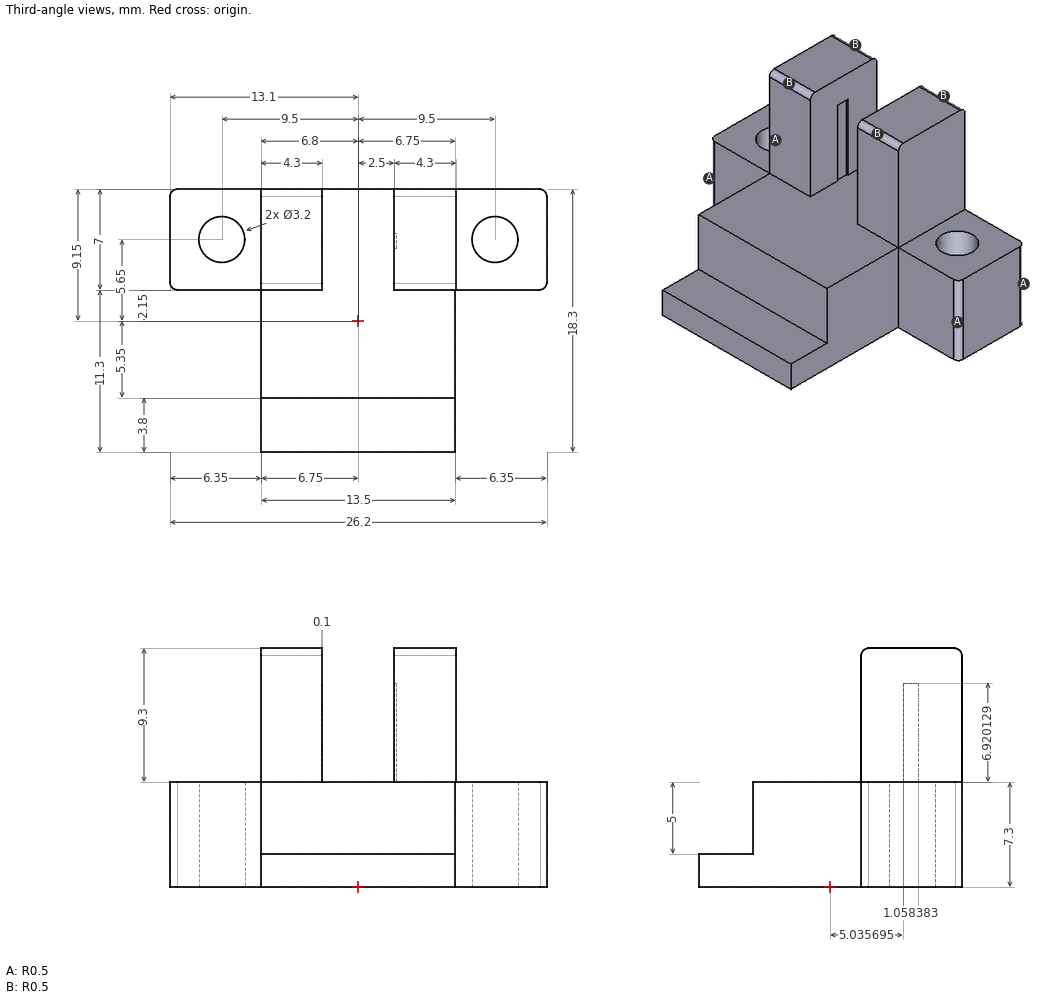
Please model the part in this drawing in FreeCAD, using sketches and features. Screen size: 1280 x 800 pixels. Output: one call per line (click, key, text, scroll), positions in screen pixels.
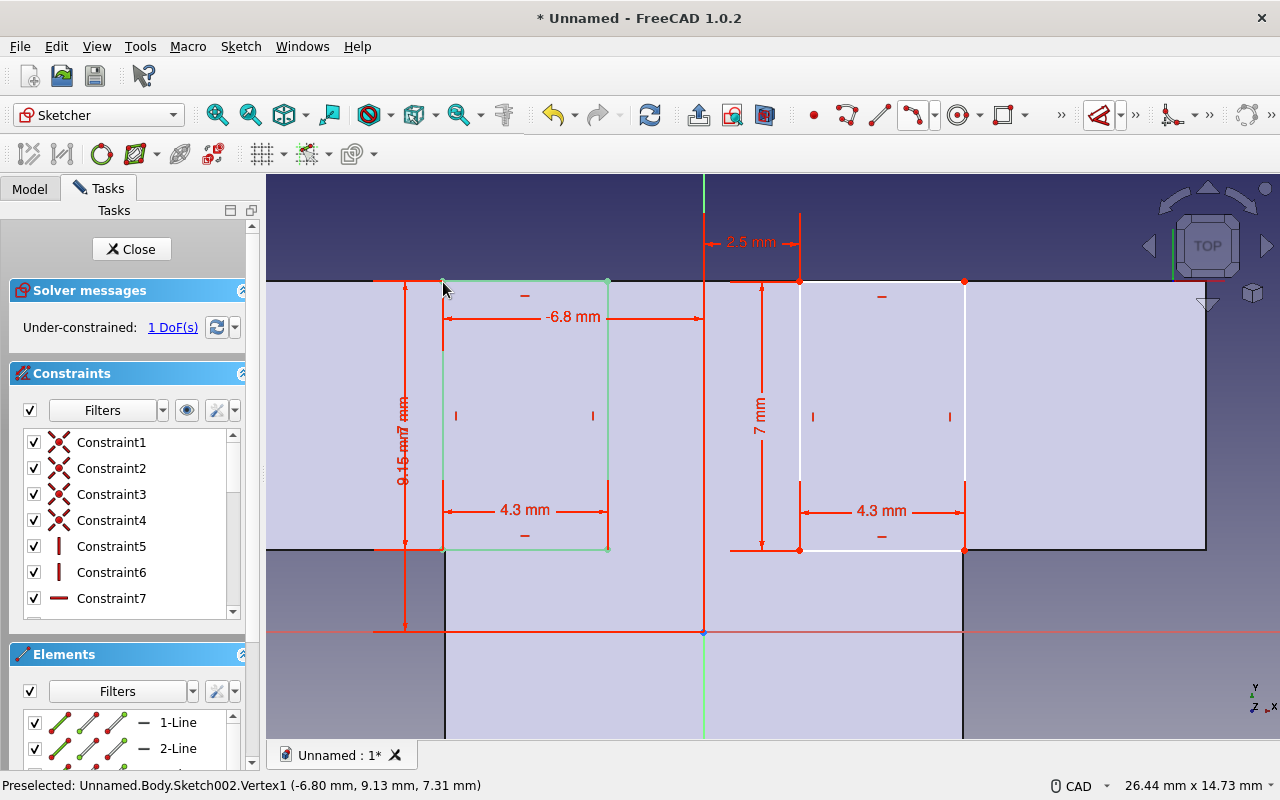
click(800, 282)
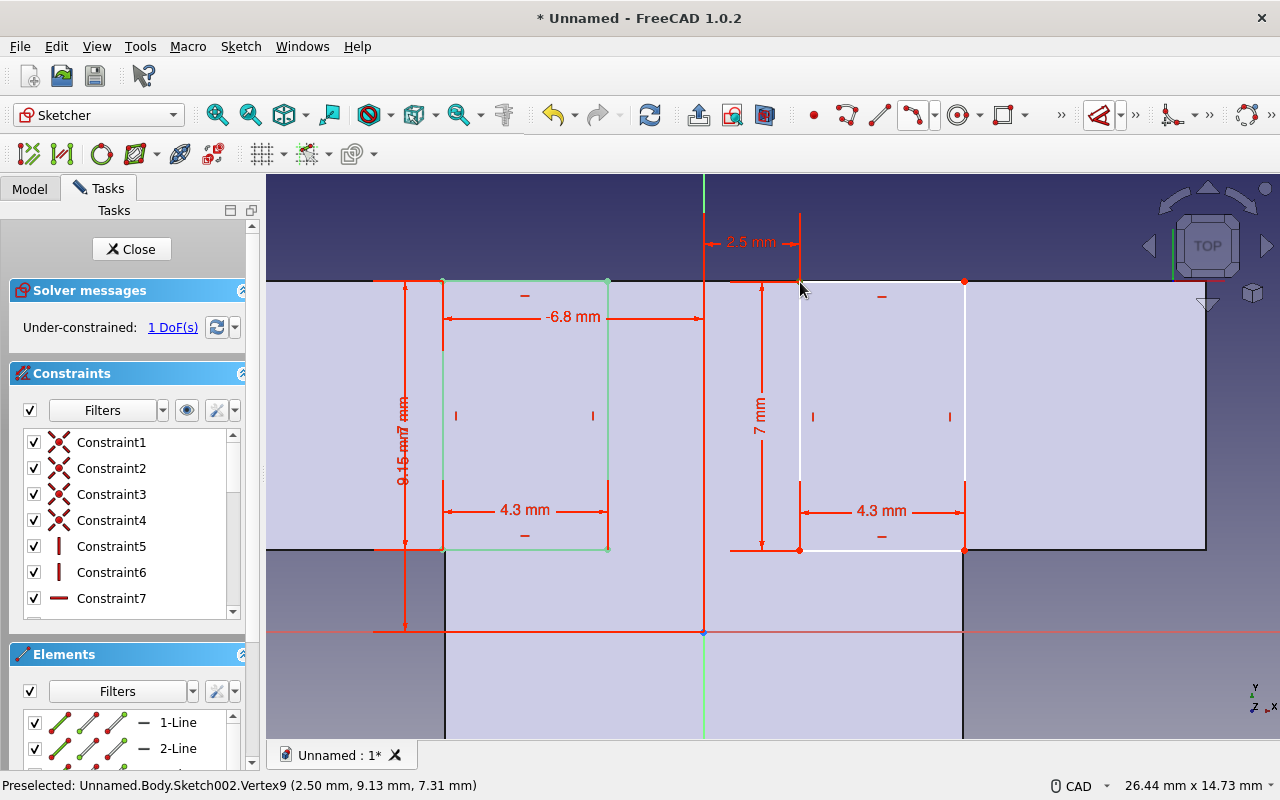
key(i)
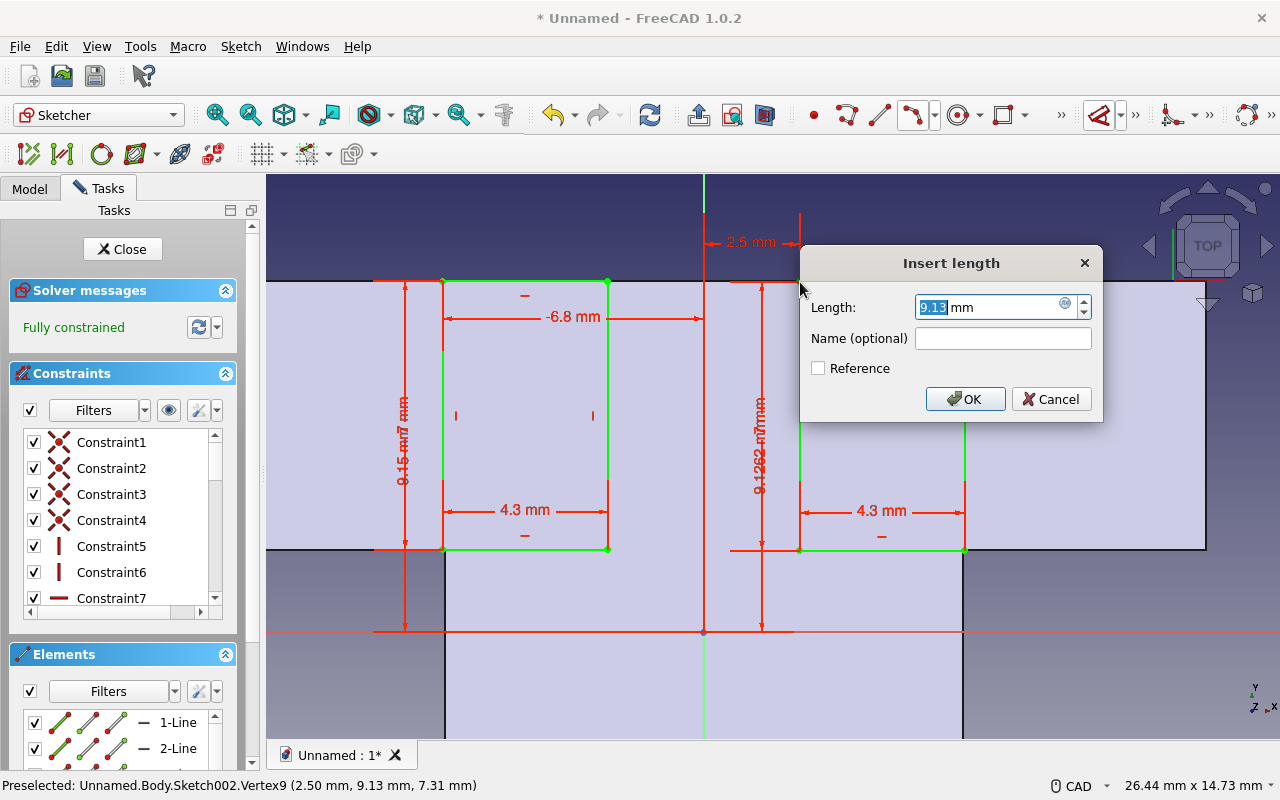
text(9.15)
key(Return)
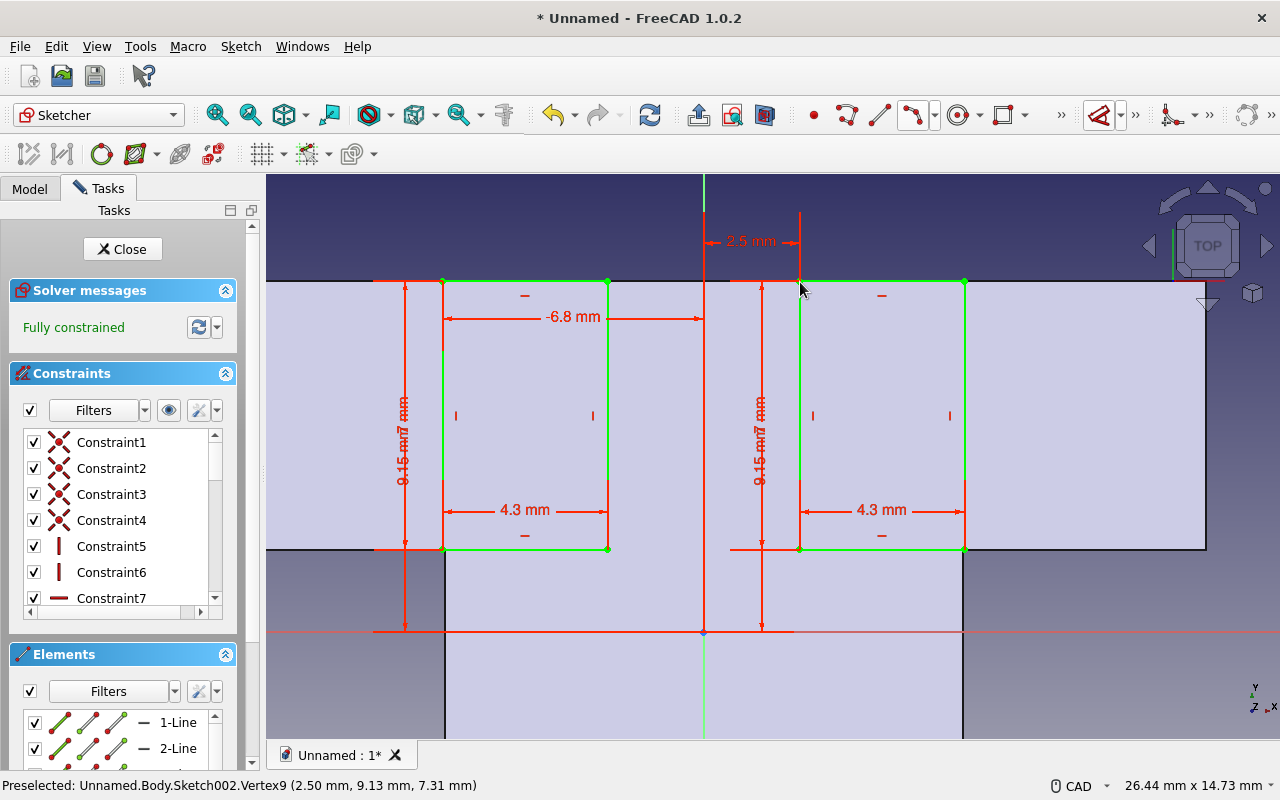
click(123, 249)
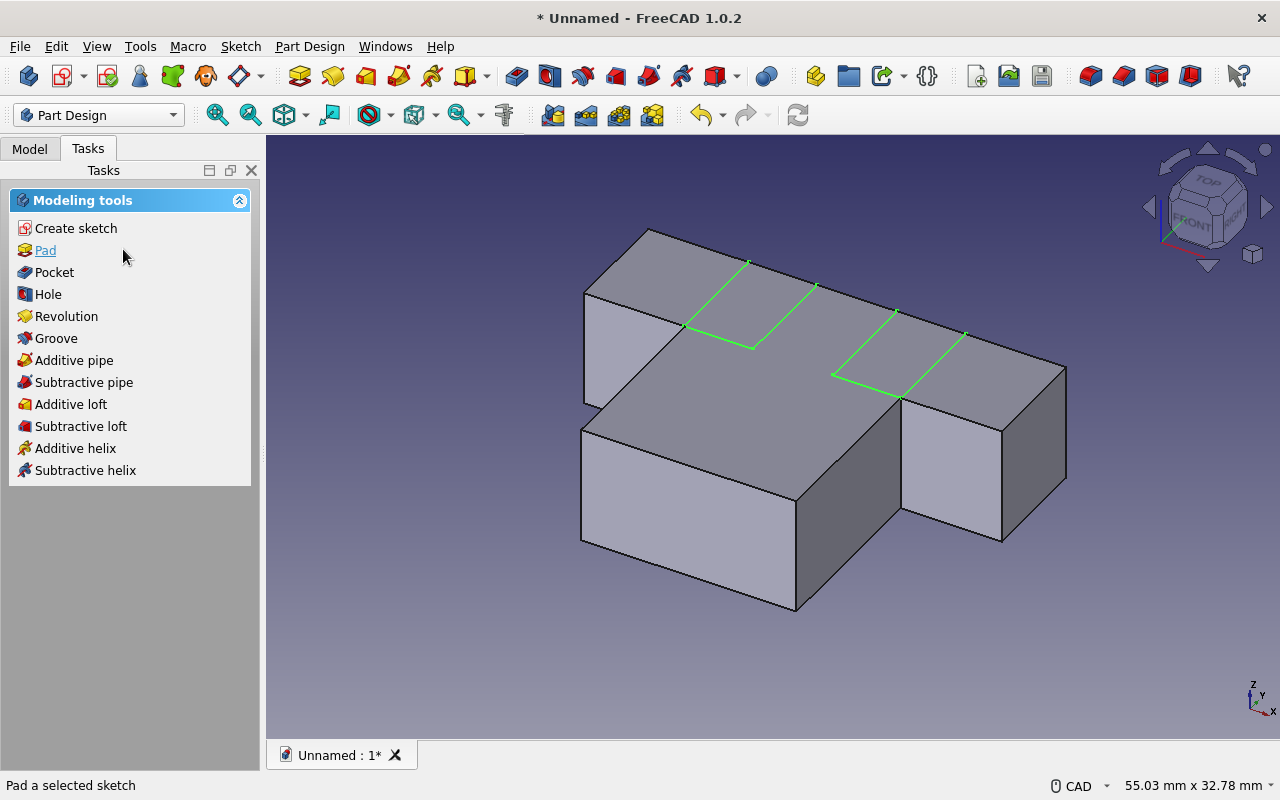
click(300, 76)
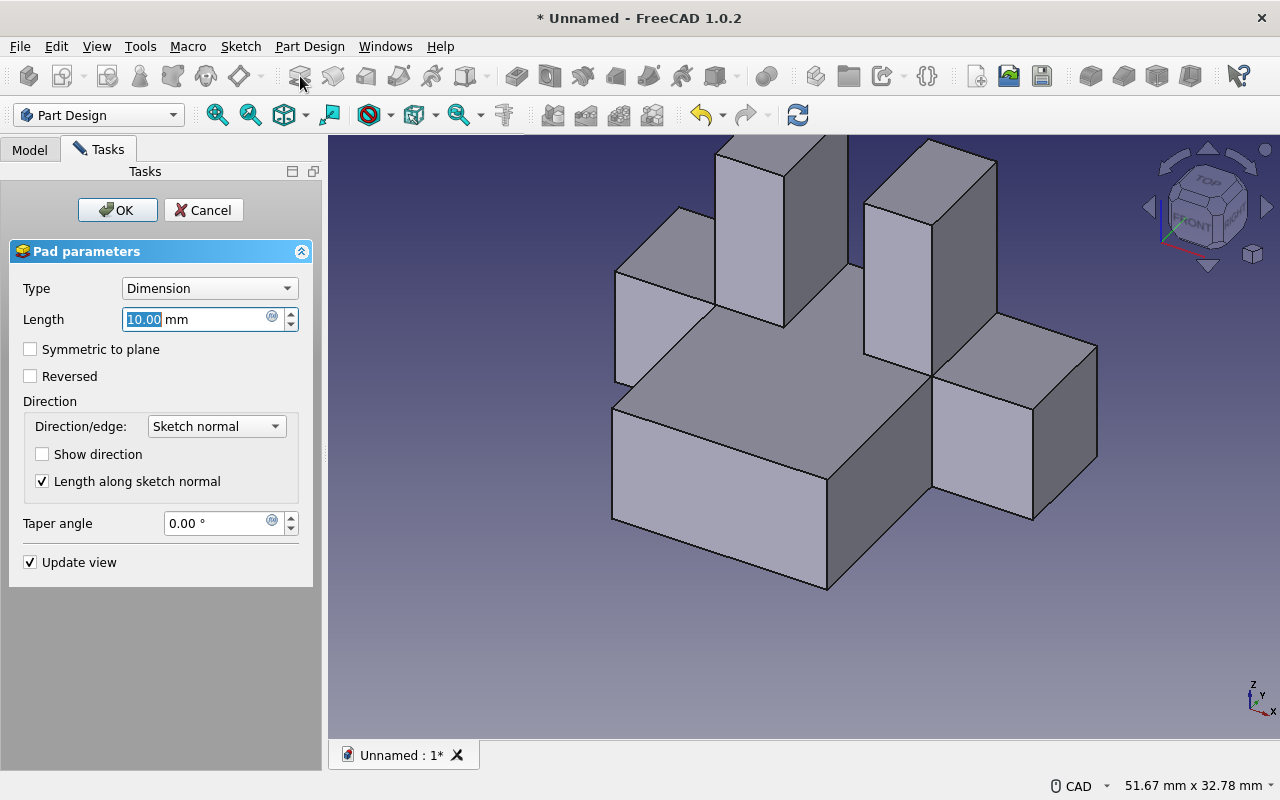
text(9.3)
key(Tab)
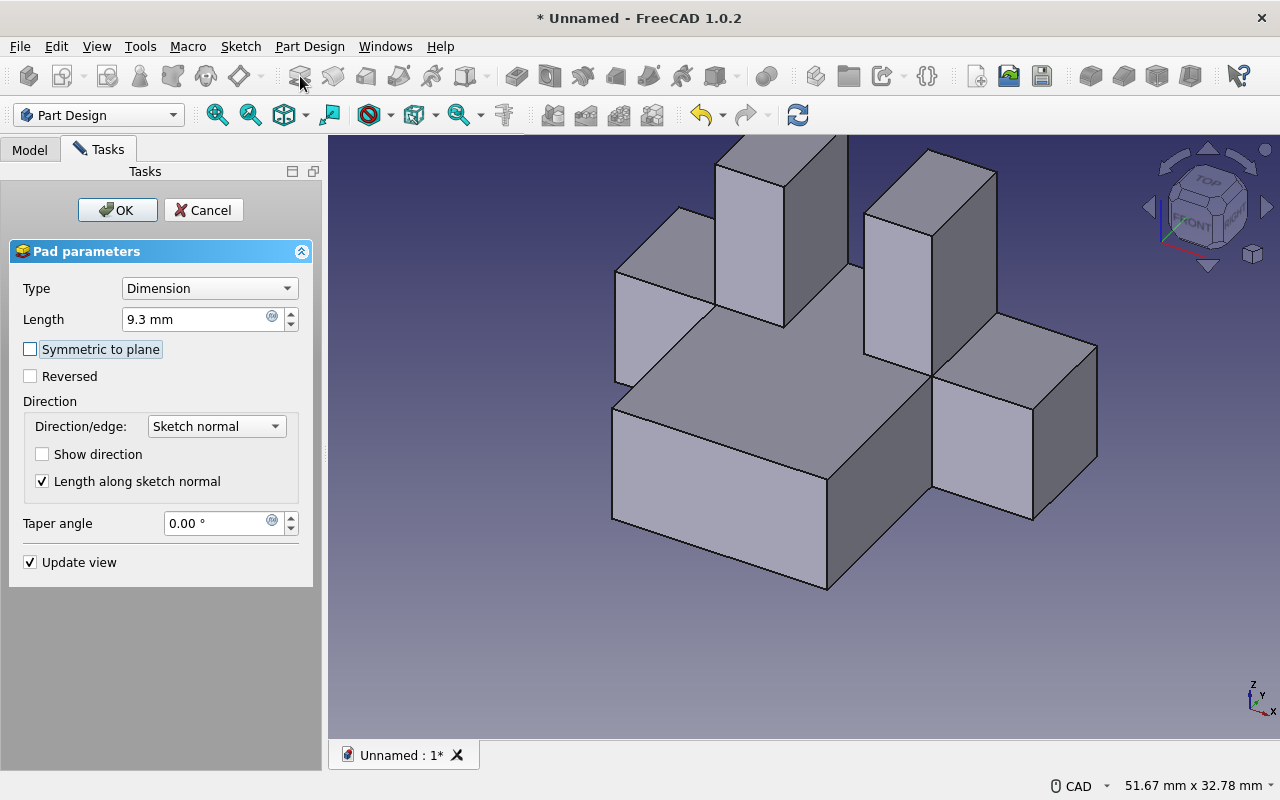
click(118, 210)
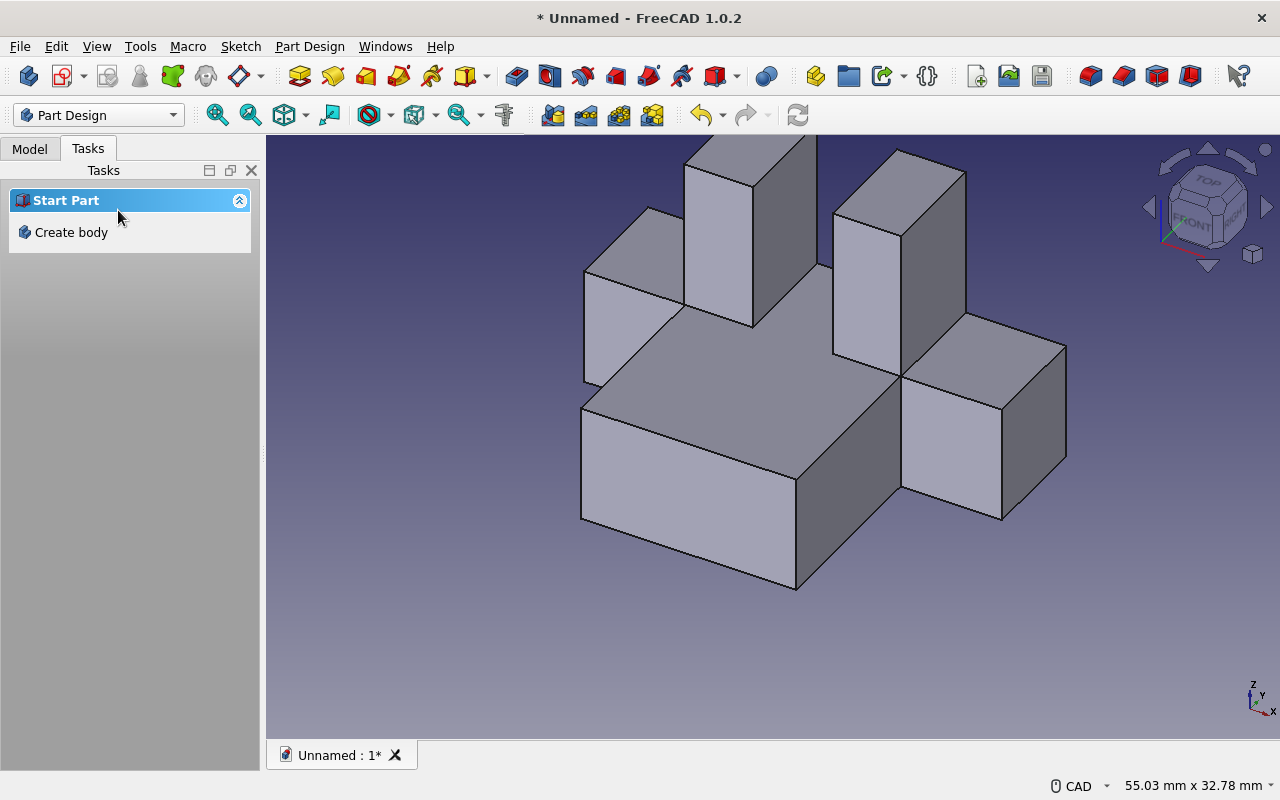
click(218, 116)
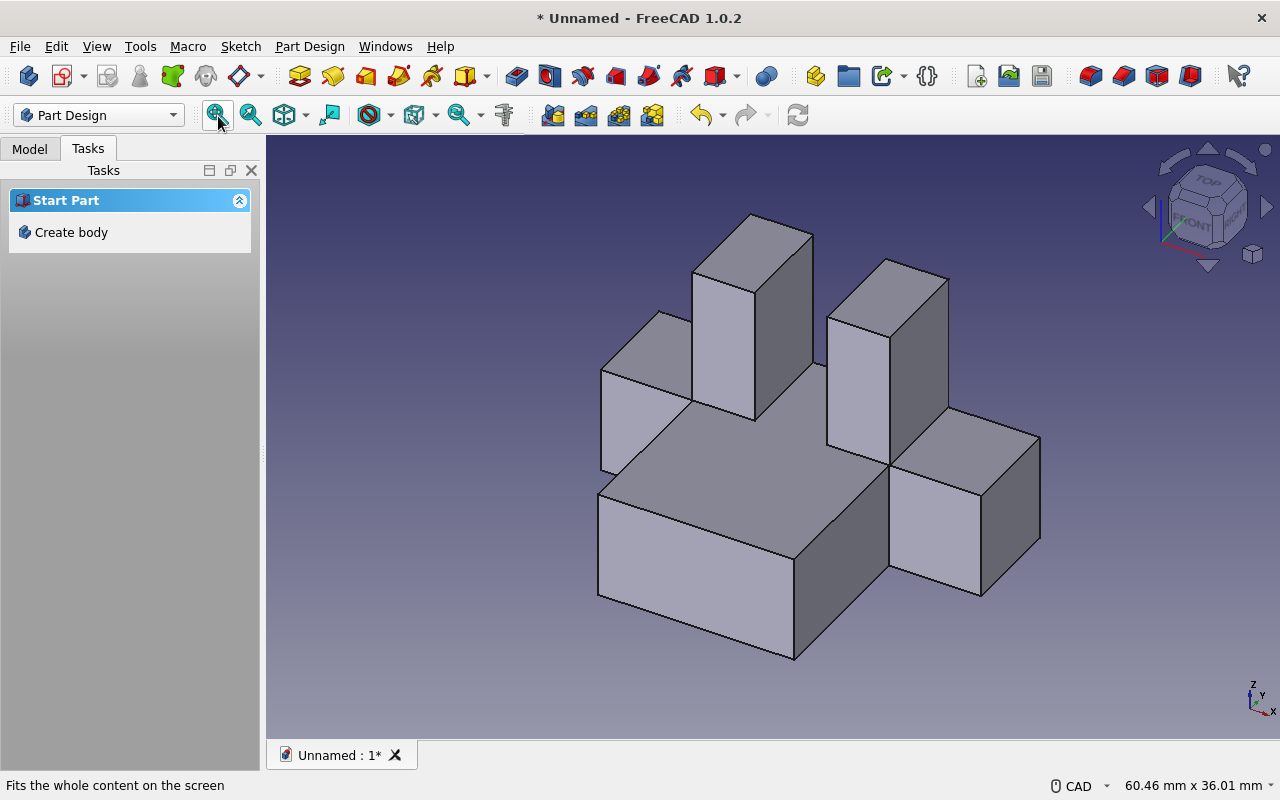
click(751, 472)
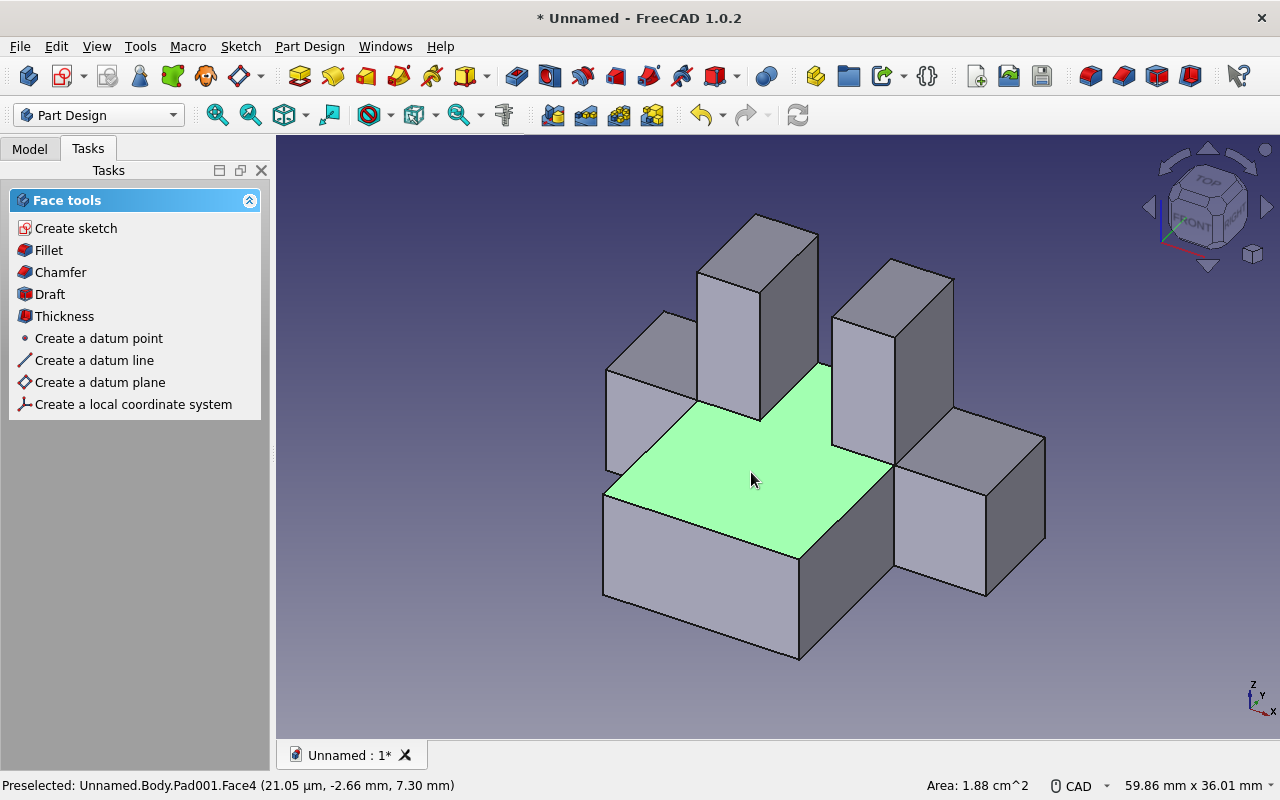
click(62, 76)